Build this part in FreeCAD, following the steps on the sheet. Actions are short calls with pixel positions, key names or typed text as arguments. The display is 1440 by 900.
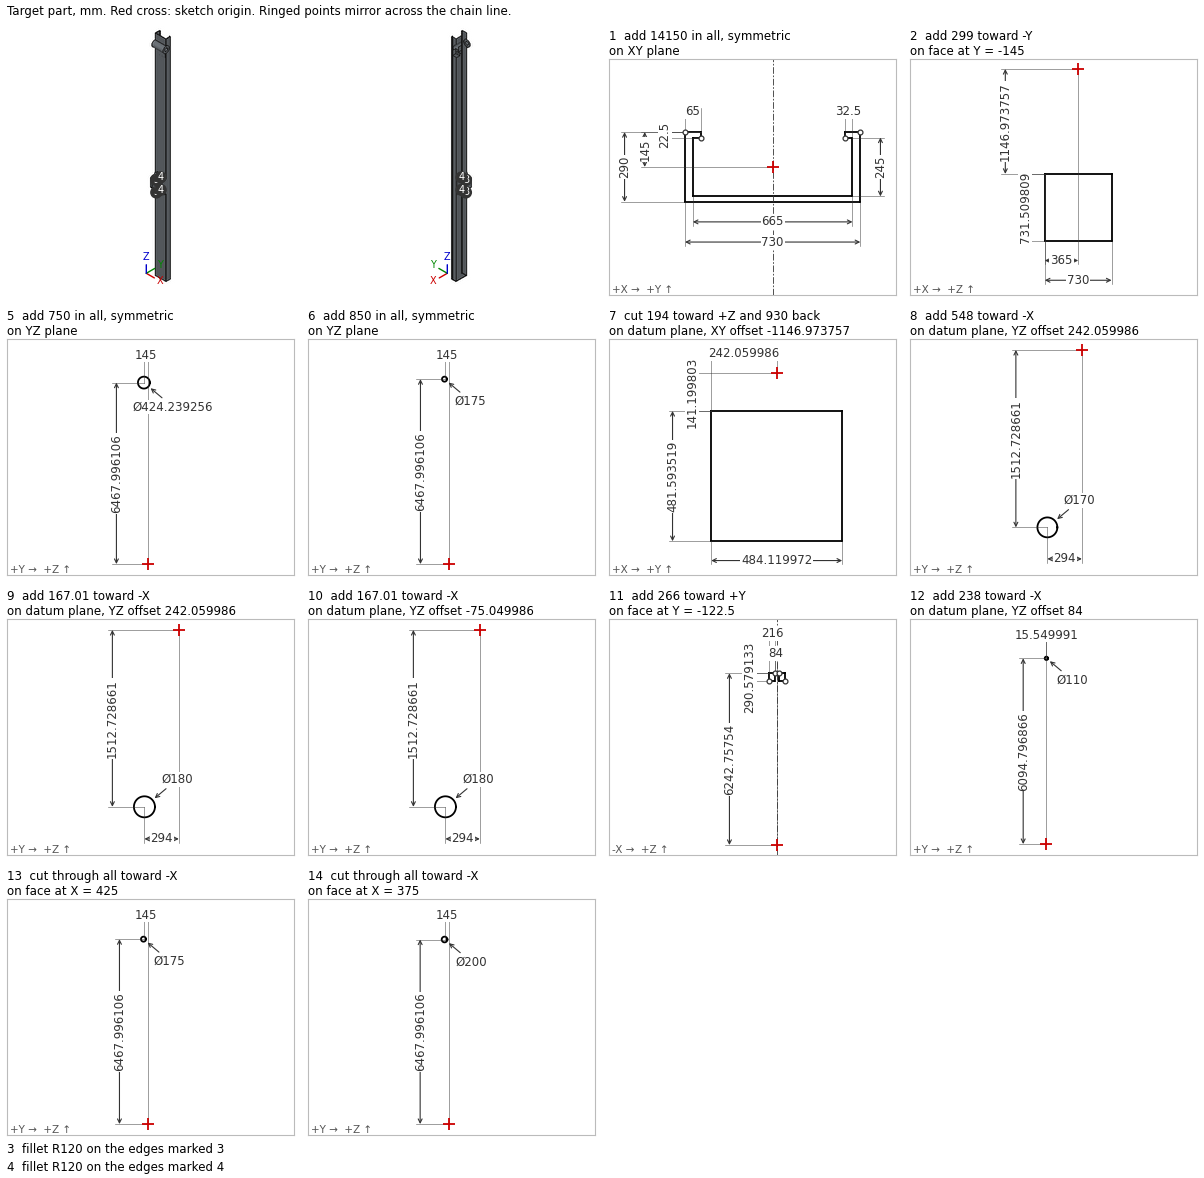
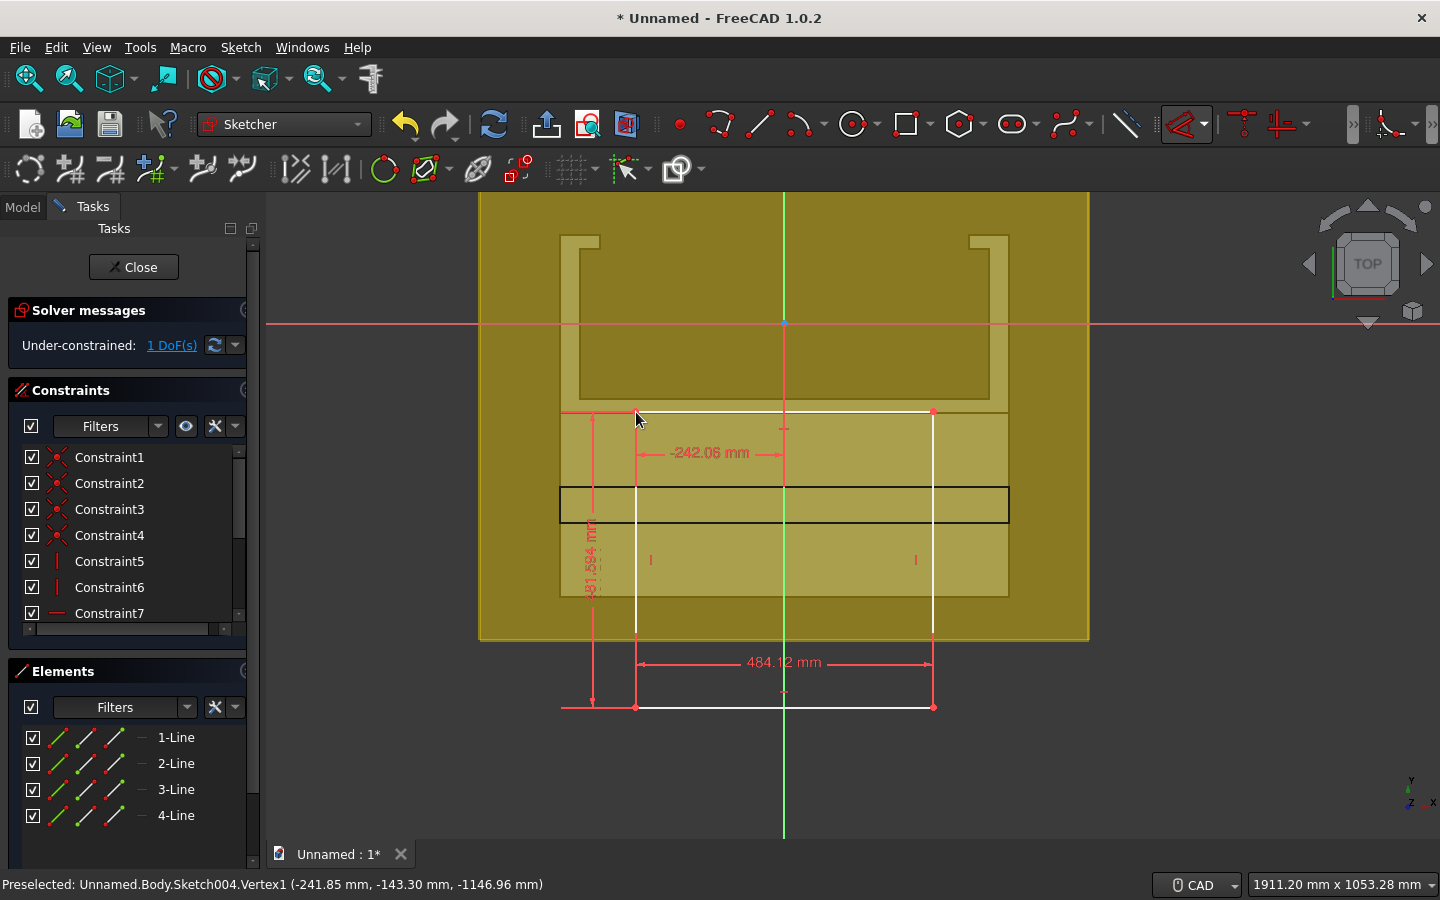
click(636, 412)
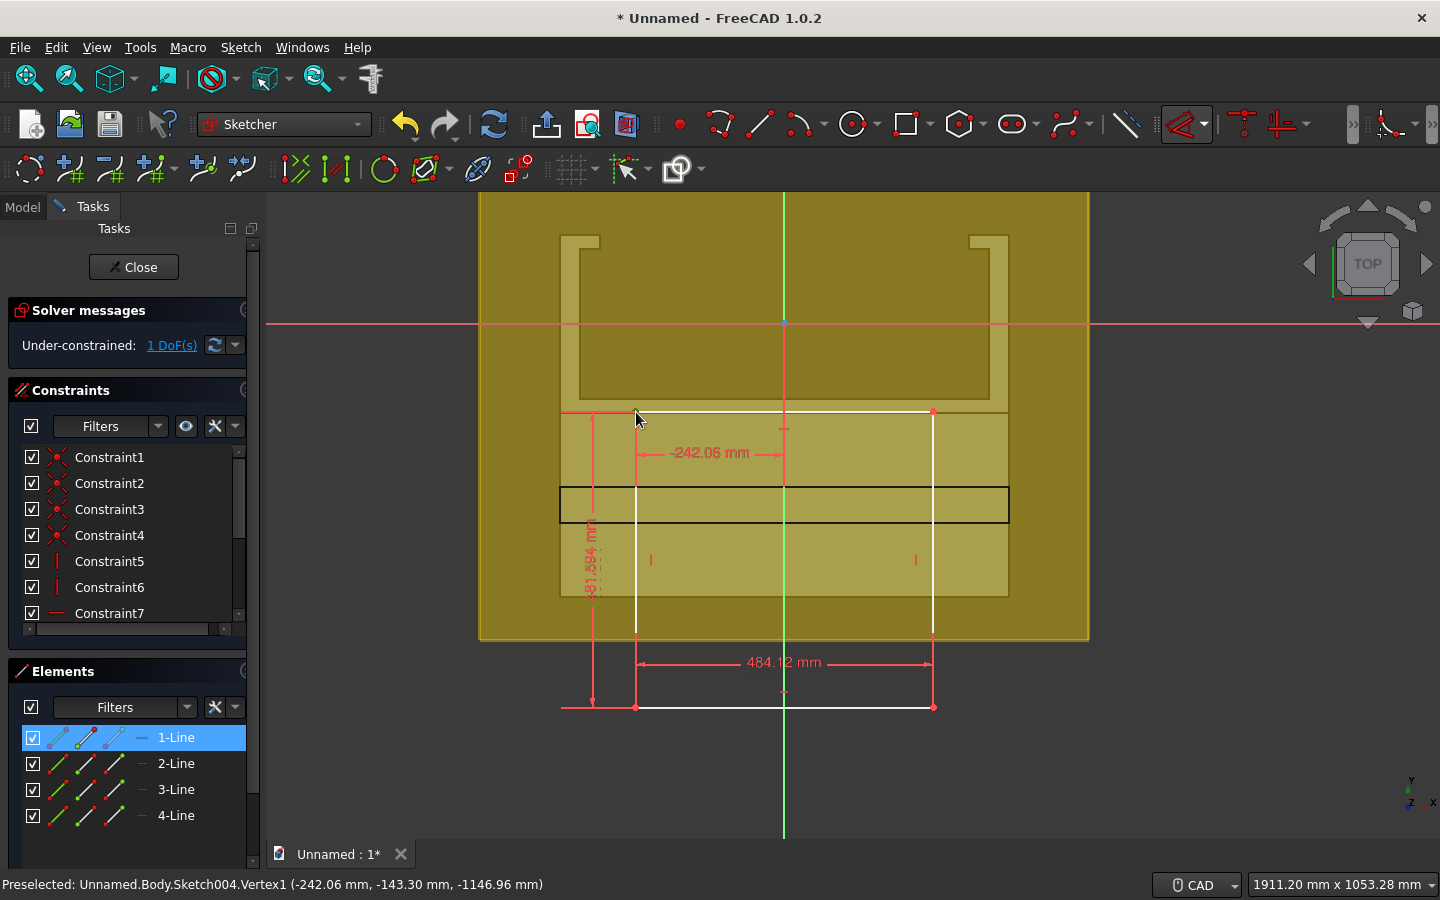
key(i)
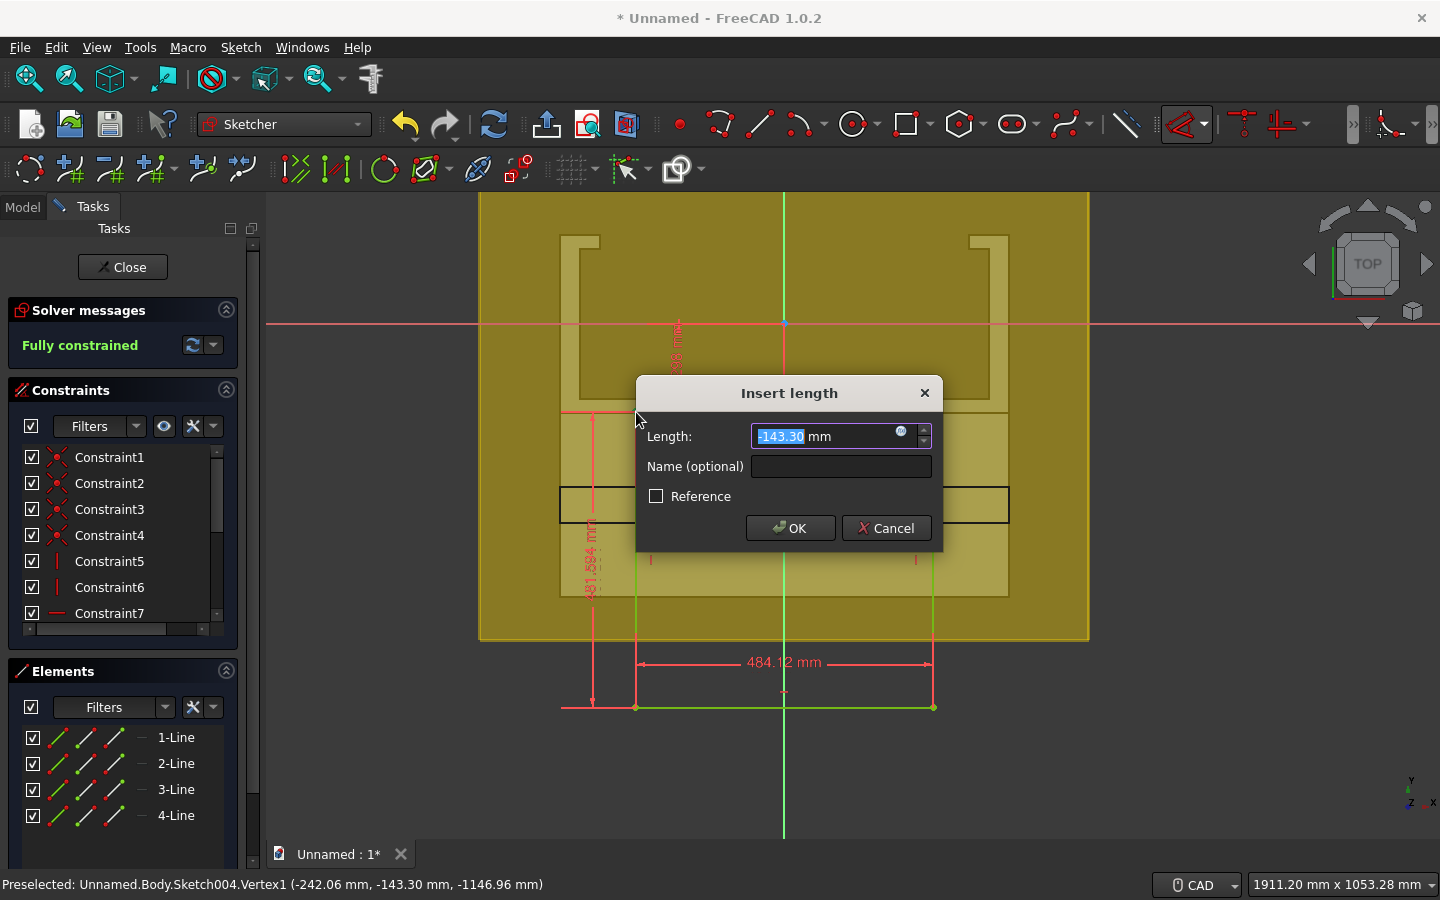
text(-141.199803)
key(Return)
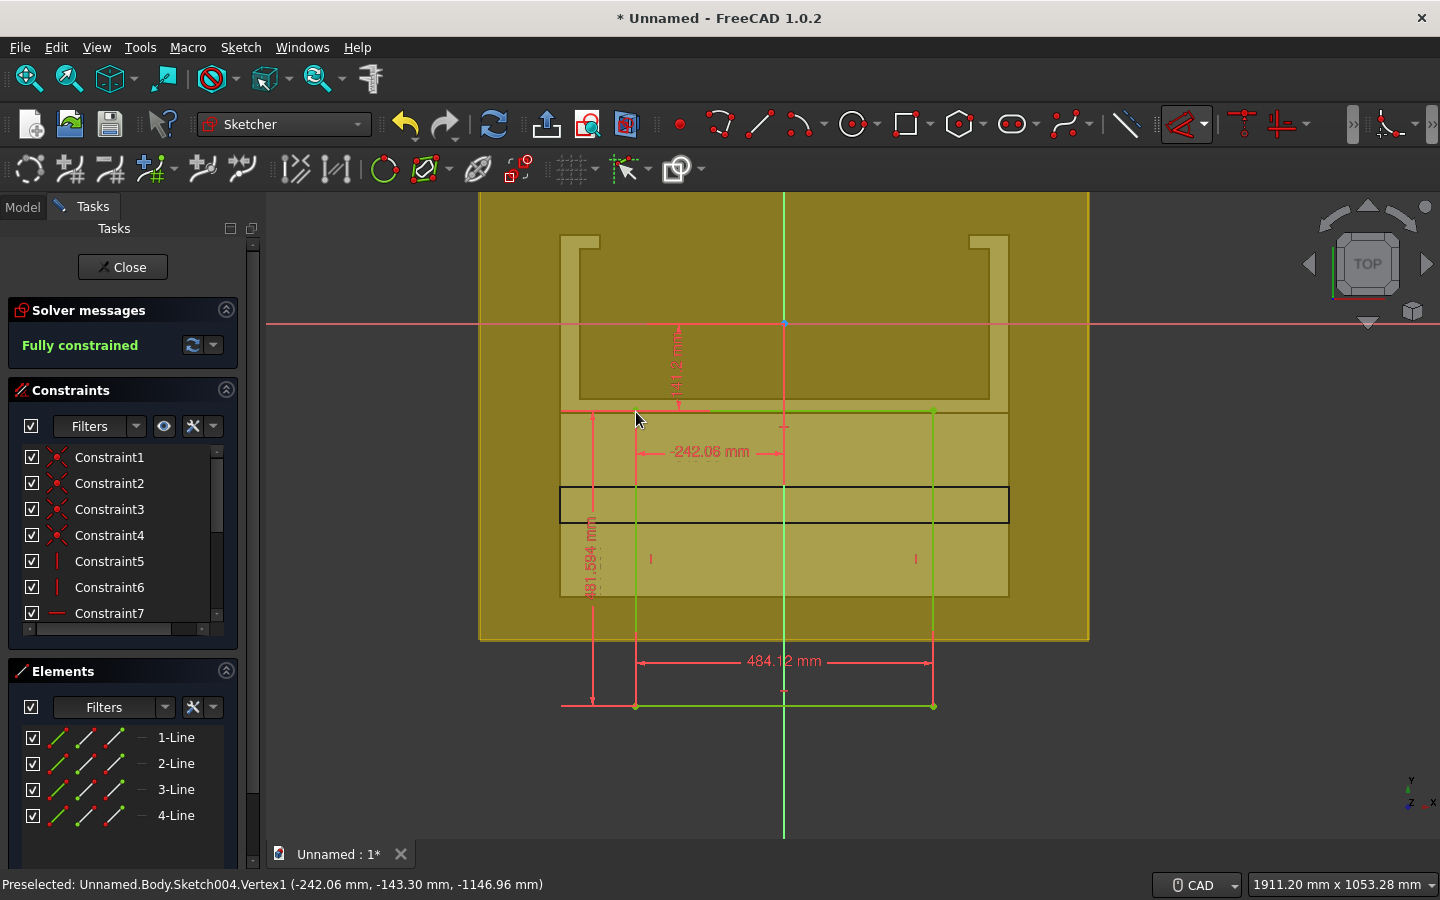
click(123, 267)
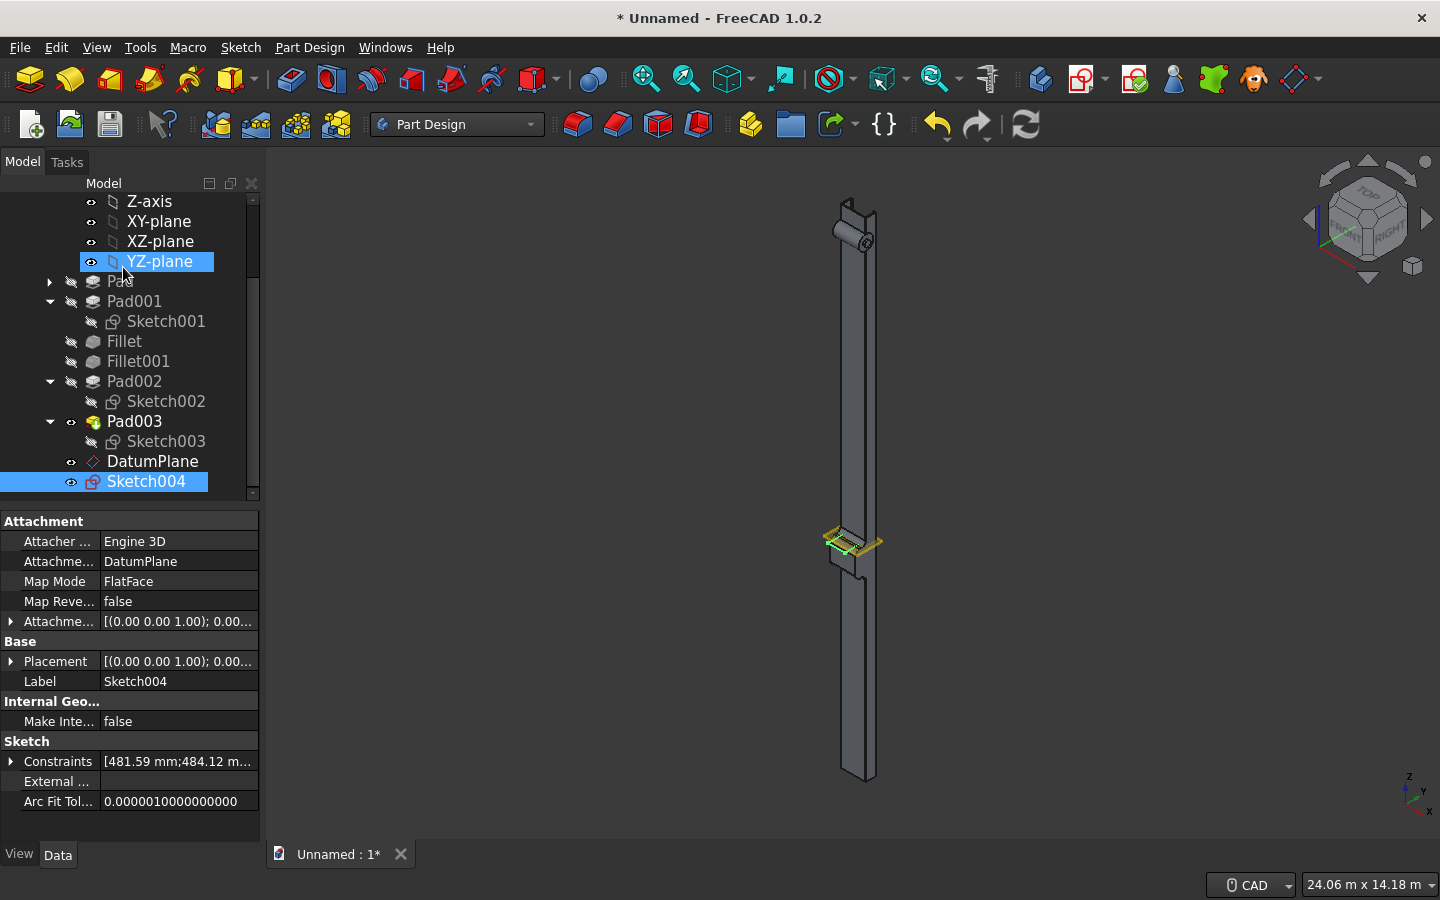
click(292, 80)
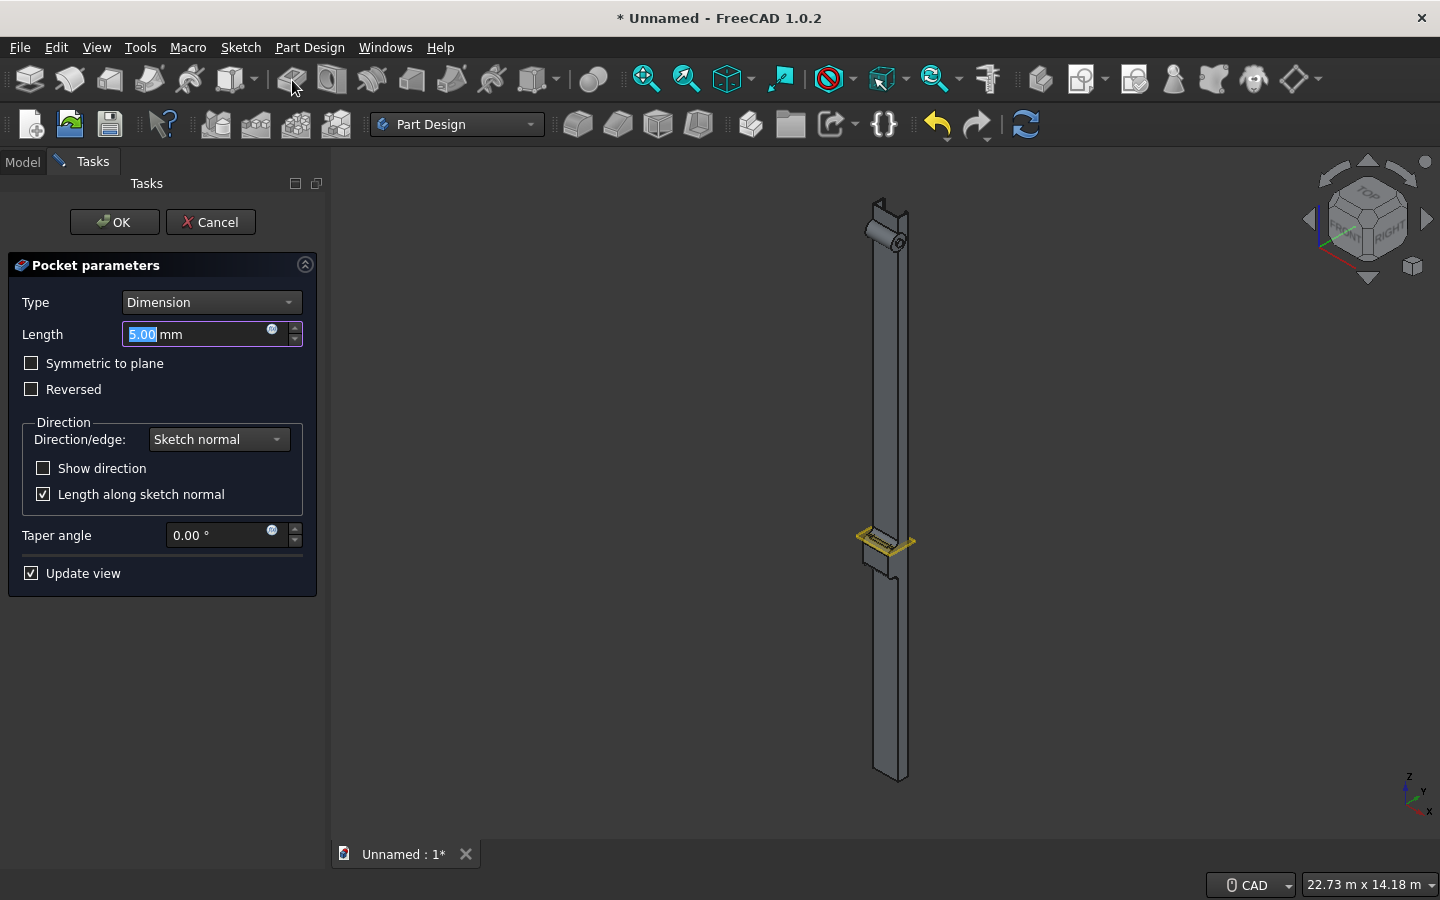
click(212, 302)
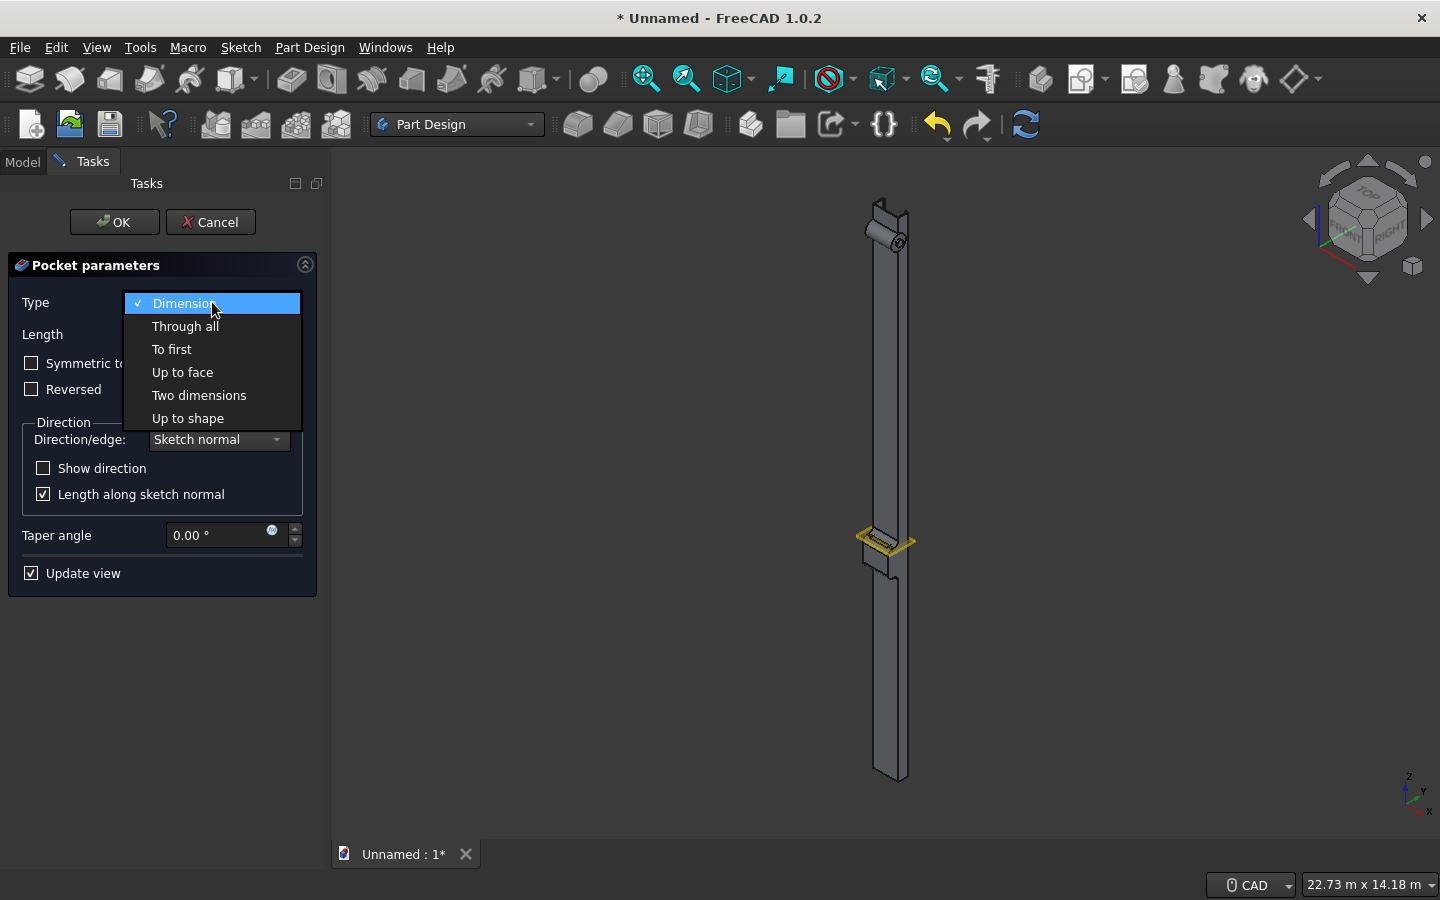
click(212, 396)